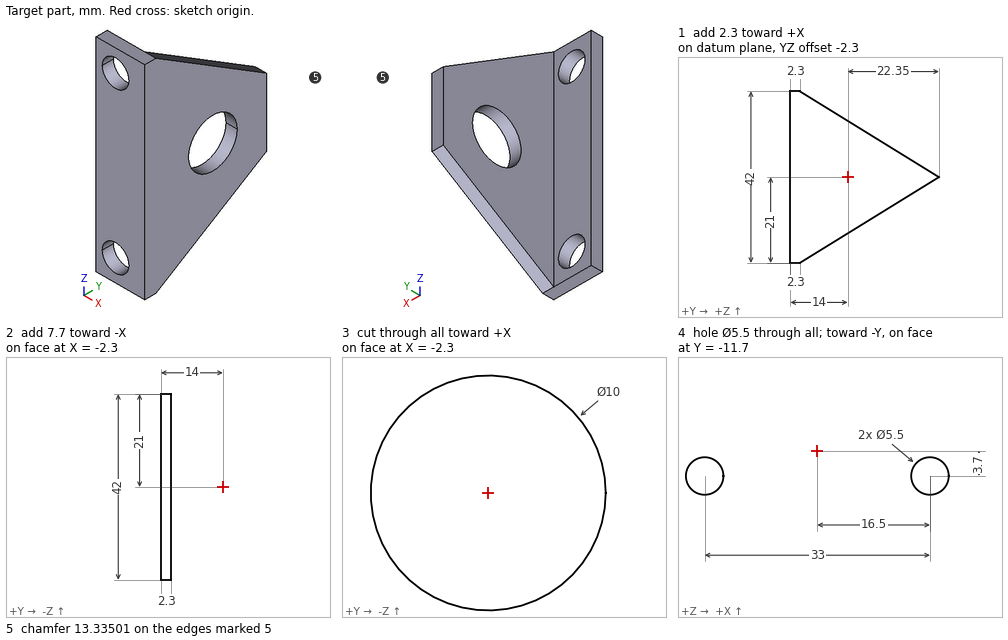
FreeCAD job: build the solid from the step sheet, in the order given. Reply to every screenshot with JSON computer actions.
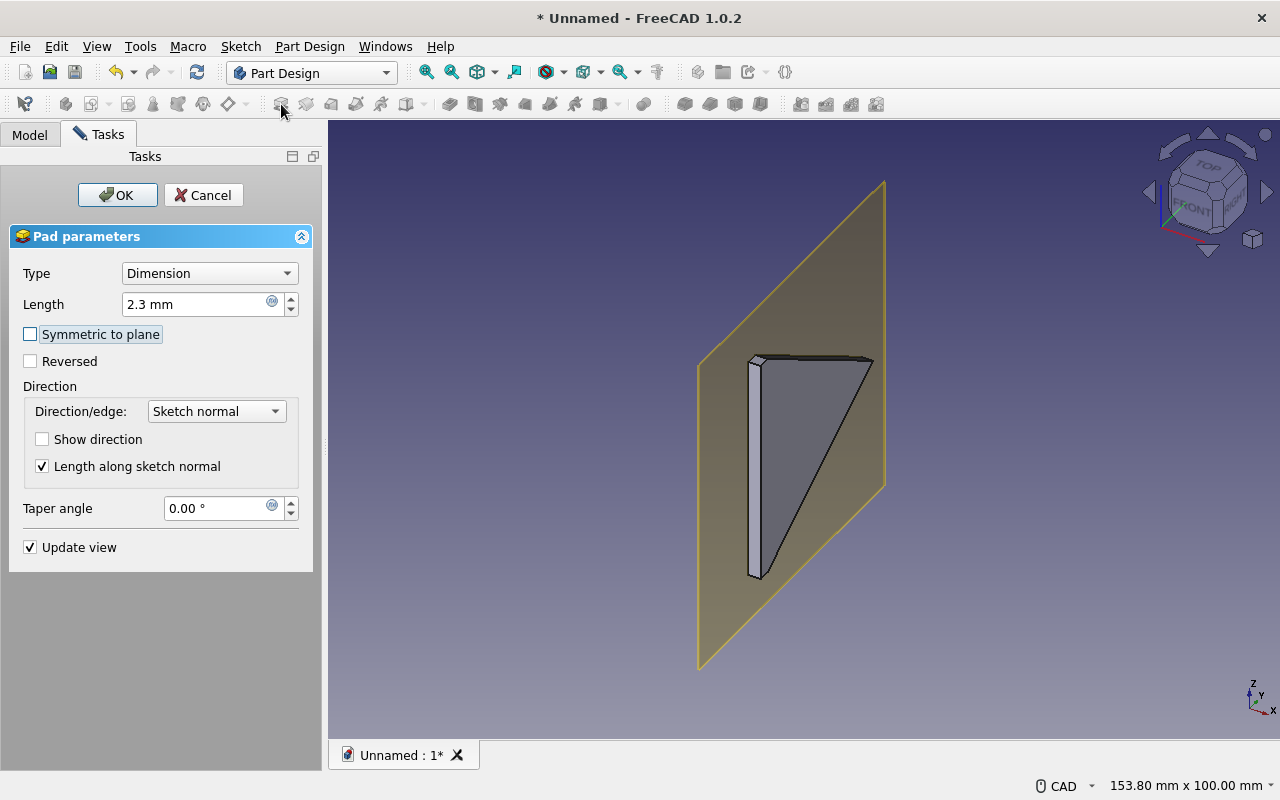
{"action": "left_click", "coordinate": [118, 195]}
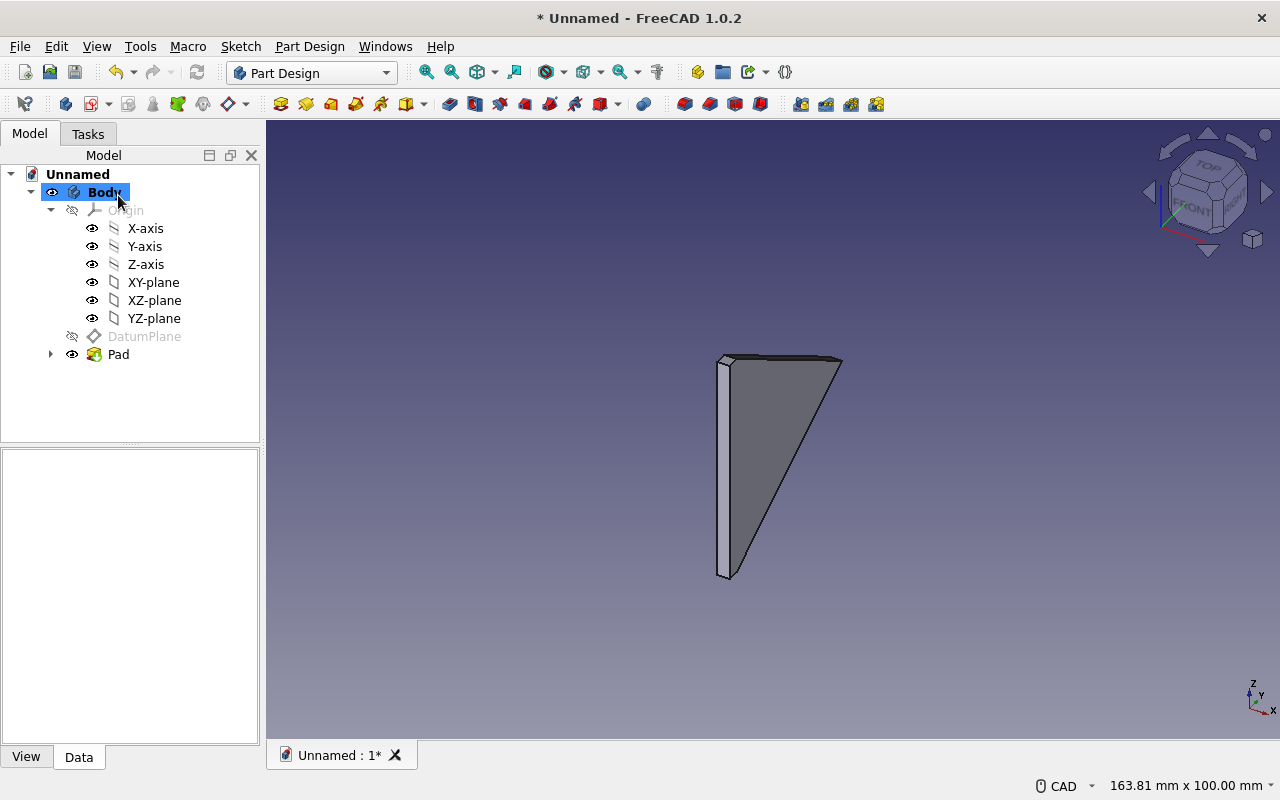
{"action": "key", "text": "6"}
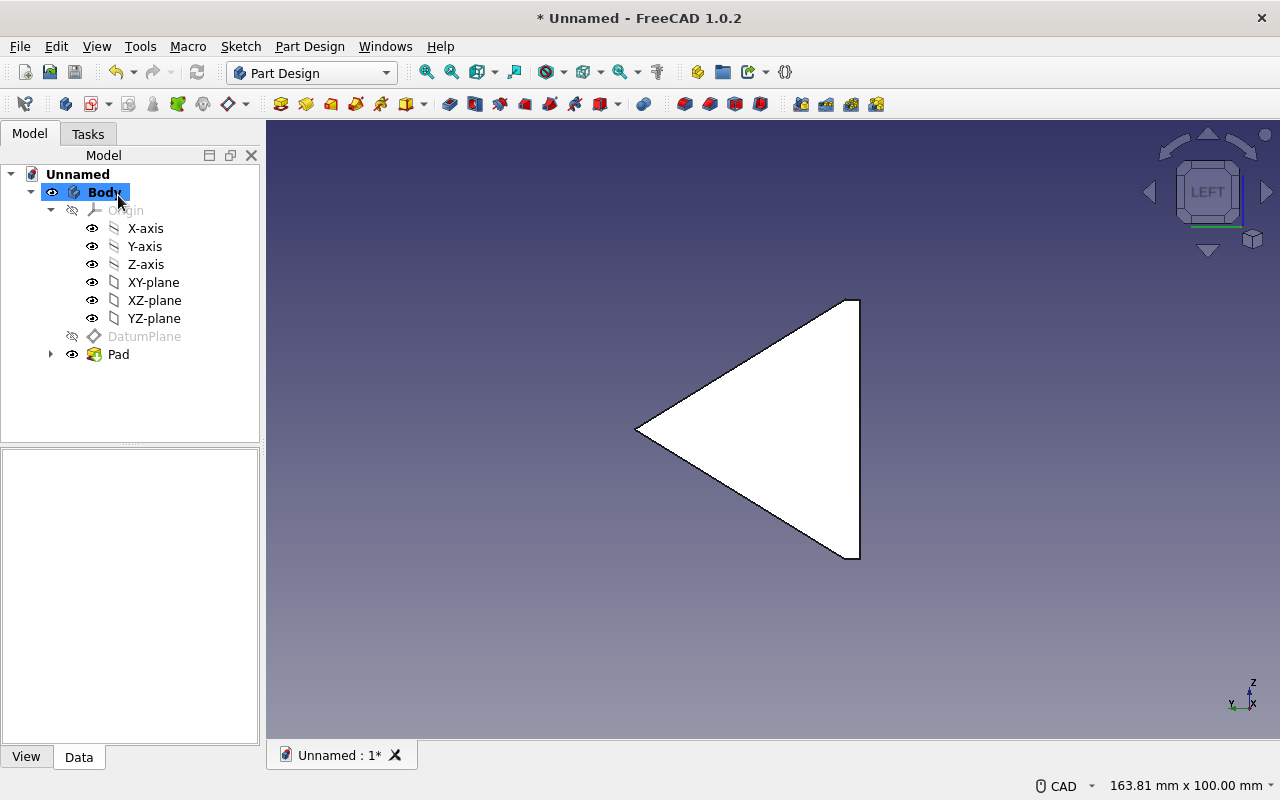
{"action": "key", "text": "v f"}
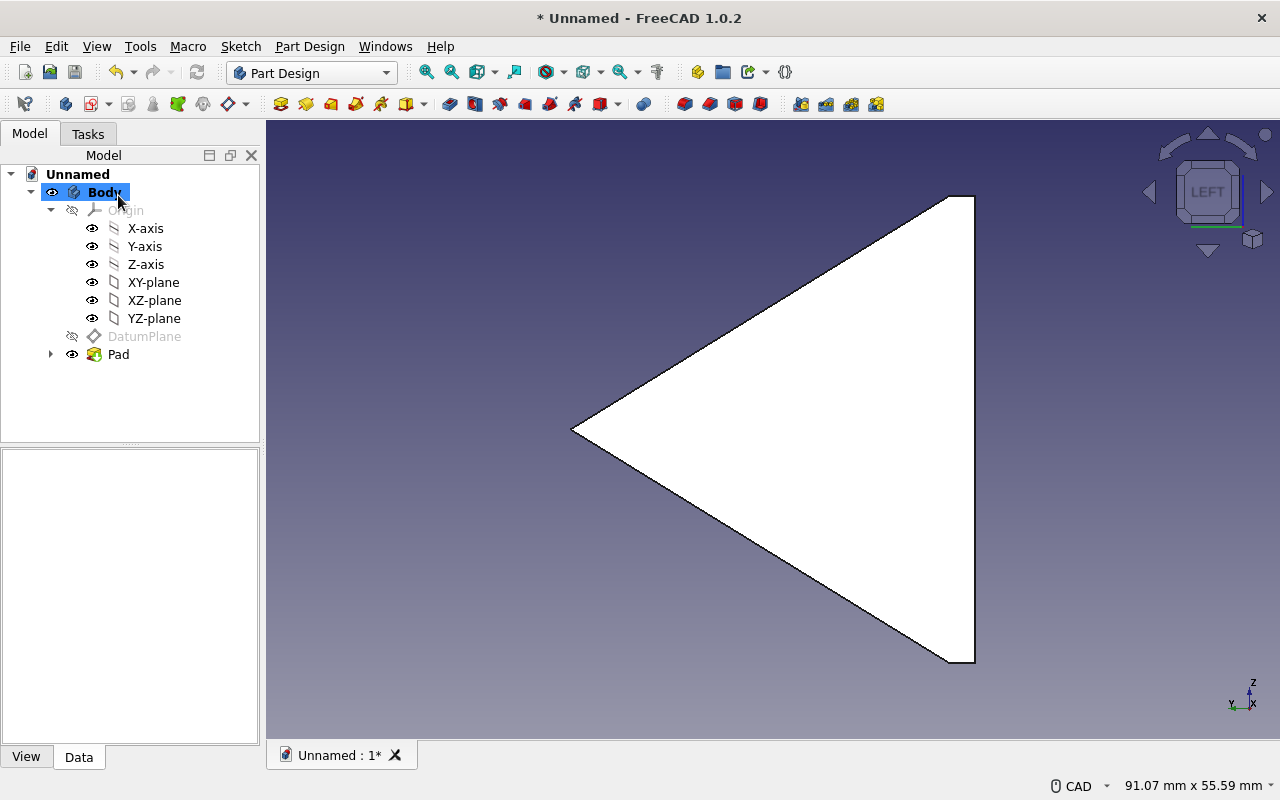
{"action": "left_click", "coordinate": [831, 428]}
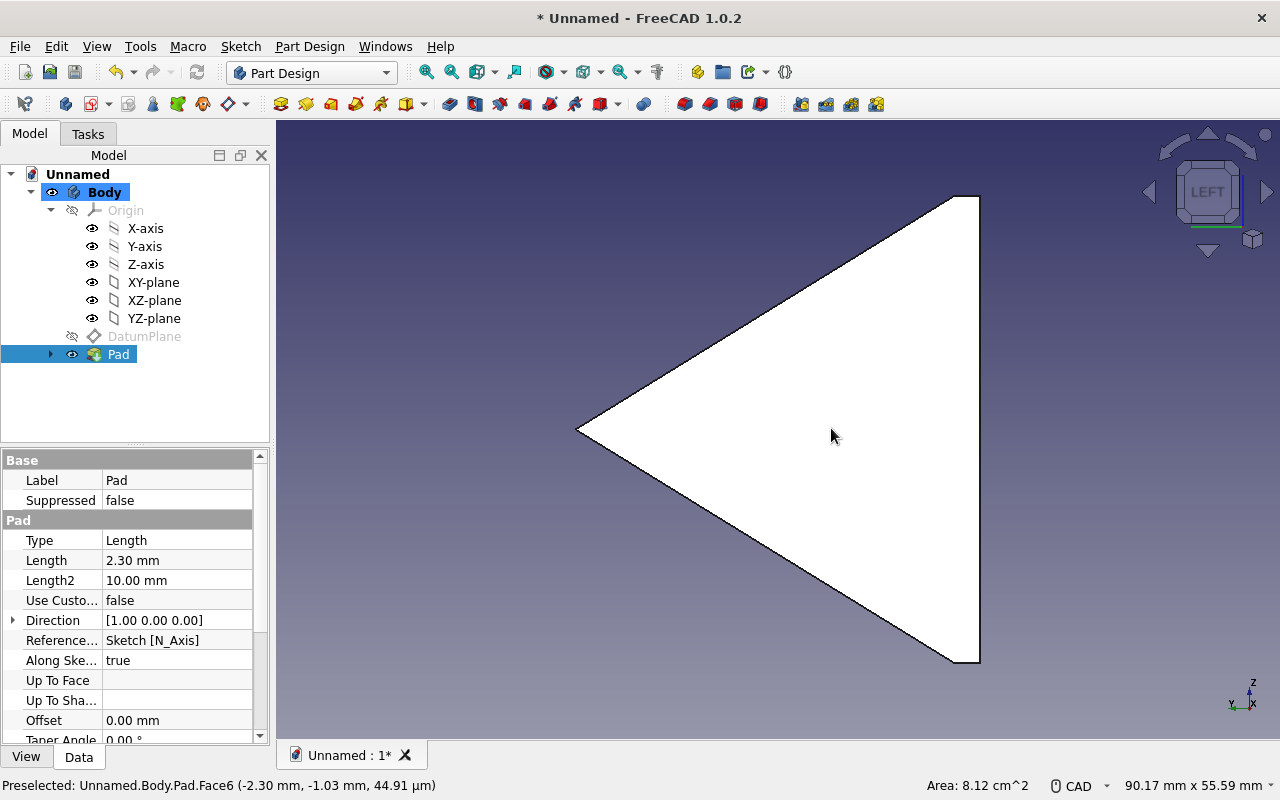
{"action": "left_click", "coordinate": [90, 104]}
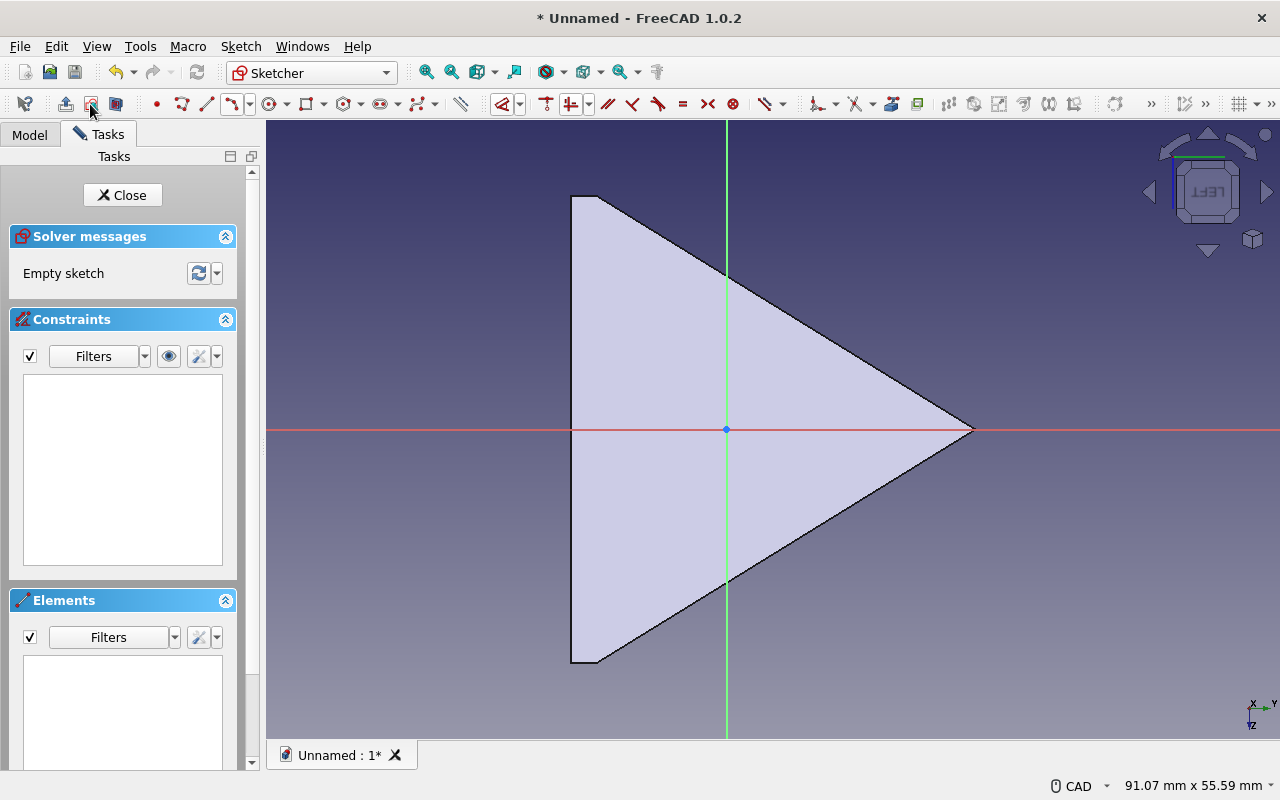
{"action": "key", "text": "g r"}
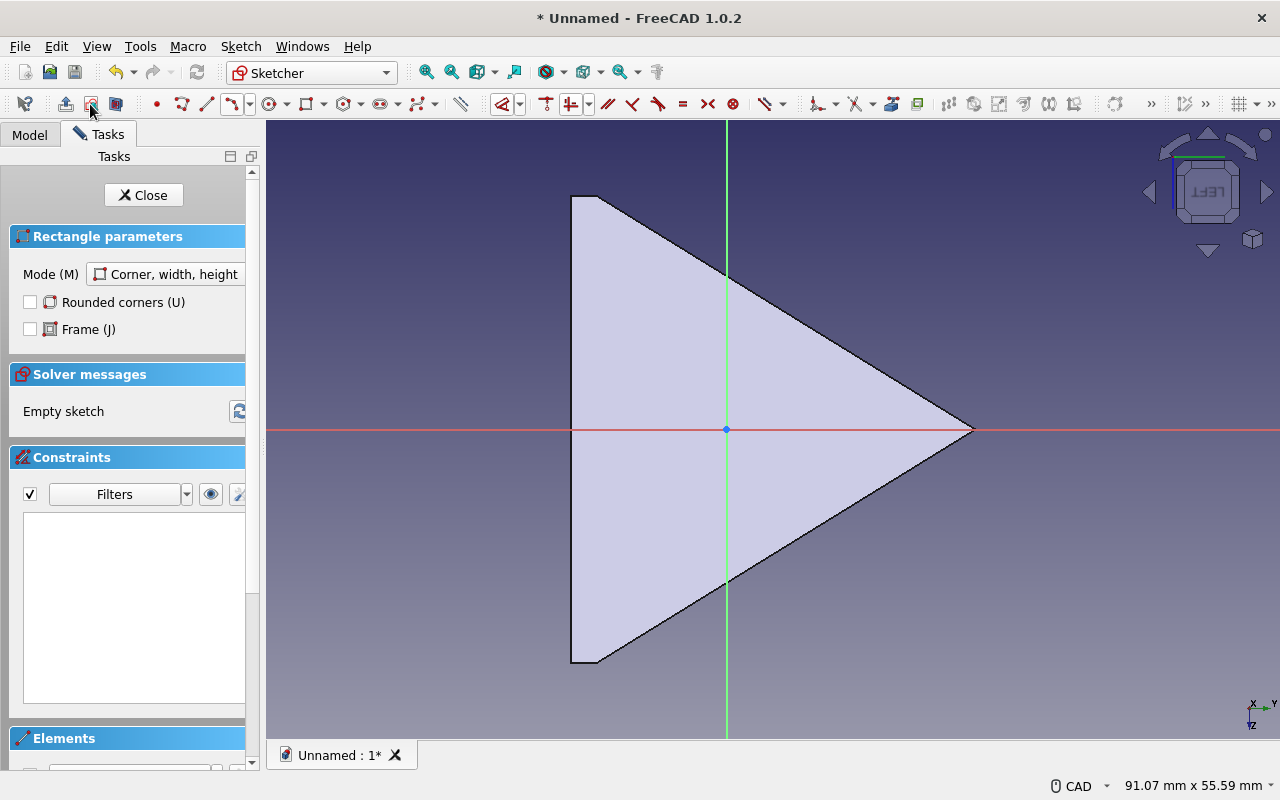
{"action": "left_click", "coordinate": [571, 196]}
{"action": "left_click", "coordinate": [596, 663]}
{"action": "key", "text": "Escape"}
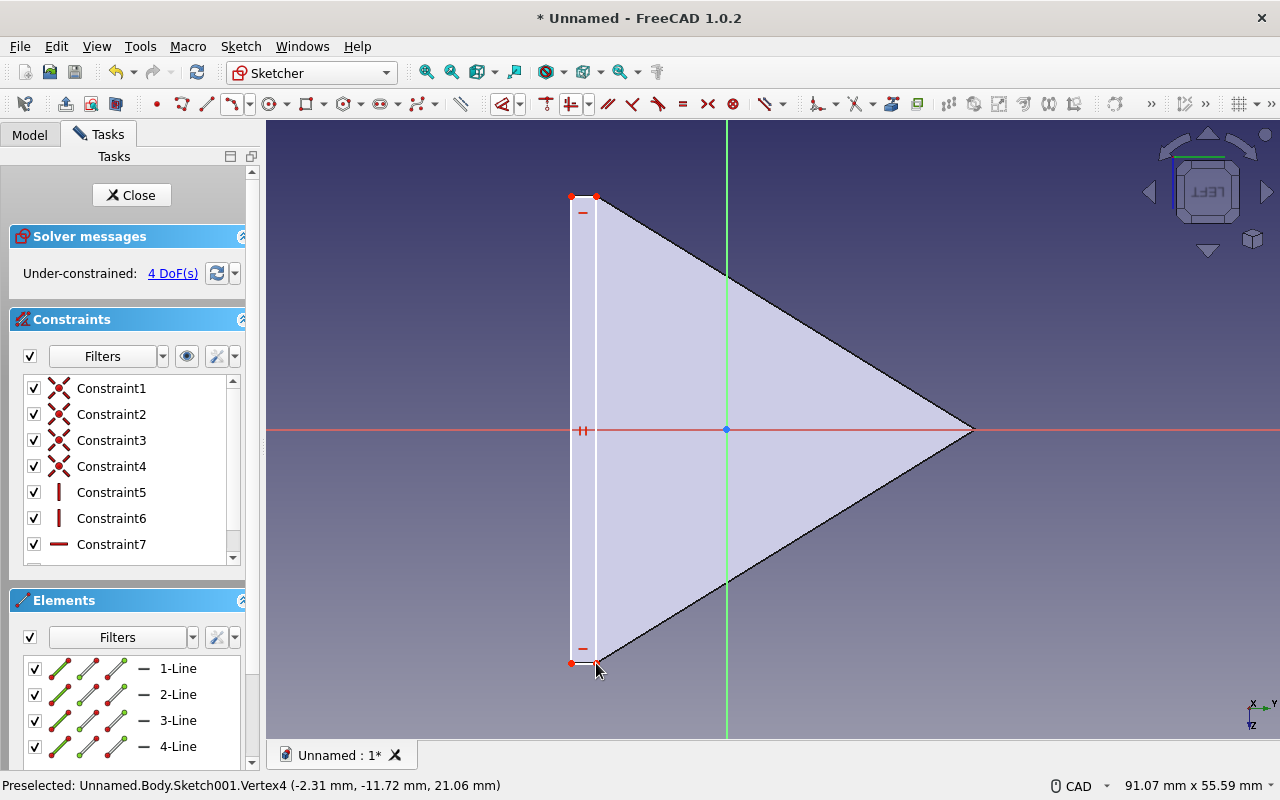
{"action": "left_click", "coordinate": [571, 337]}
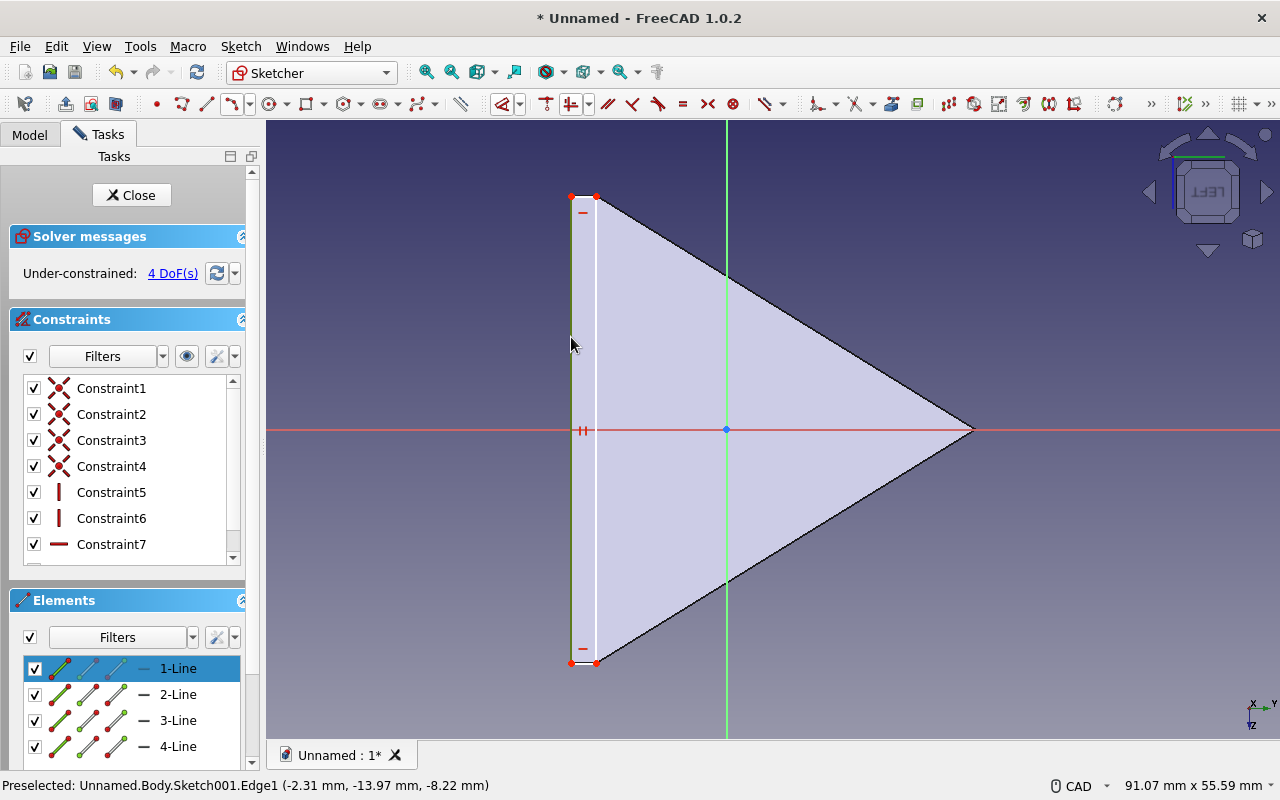
{"action": "key", "text": "i"}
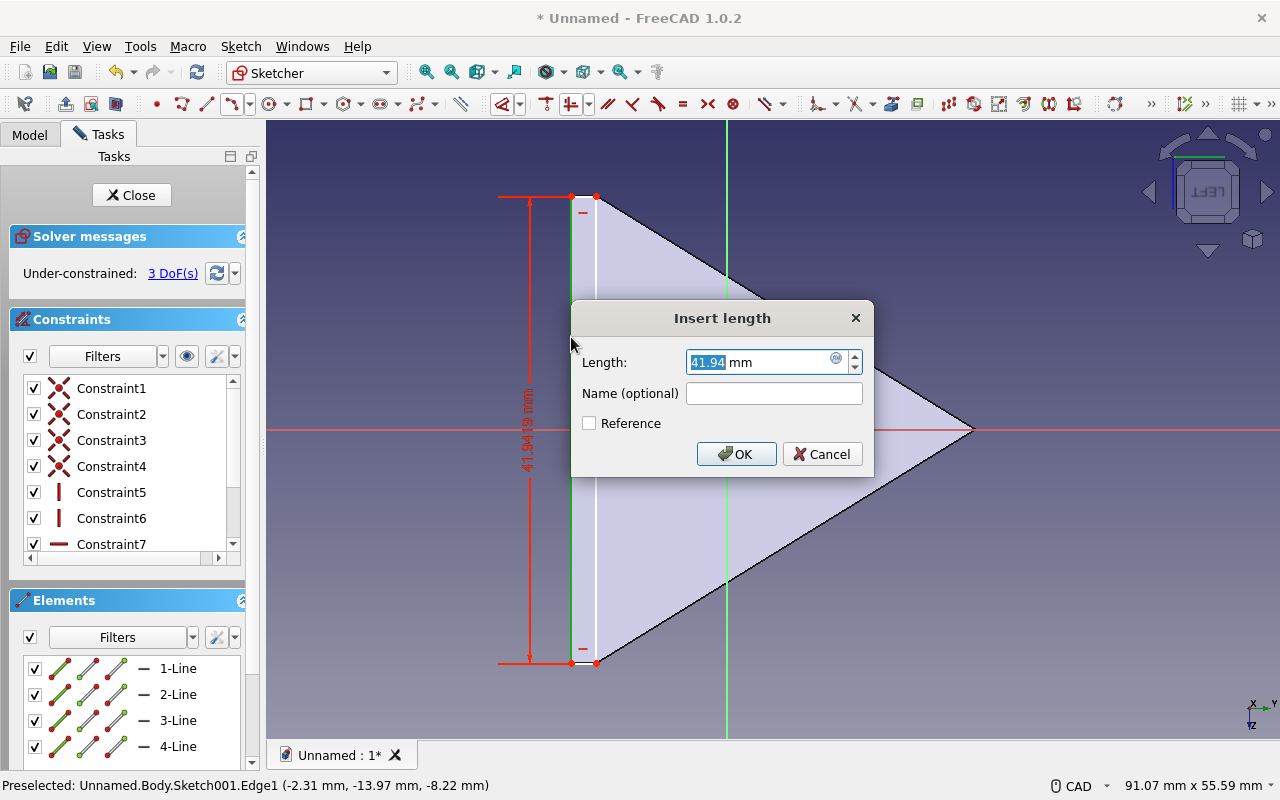
{"action": "type", "text": "42"}
{"action": "key", "text": "Return"}